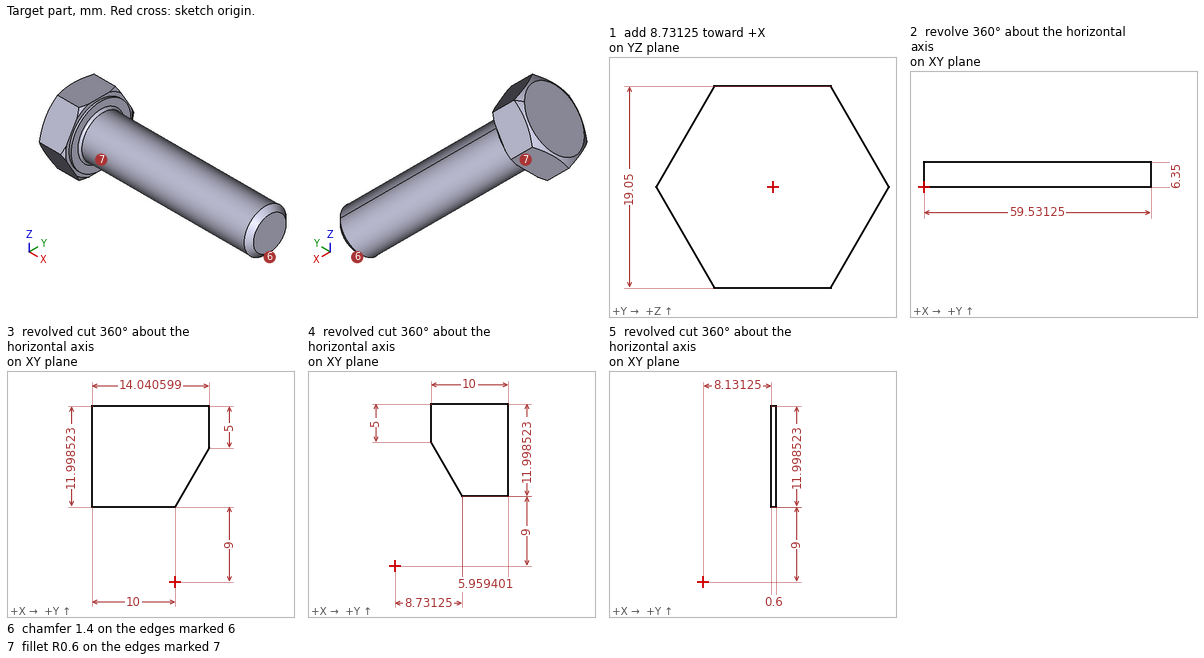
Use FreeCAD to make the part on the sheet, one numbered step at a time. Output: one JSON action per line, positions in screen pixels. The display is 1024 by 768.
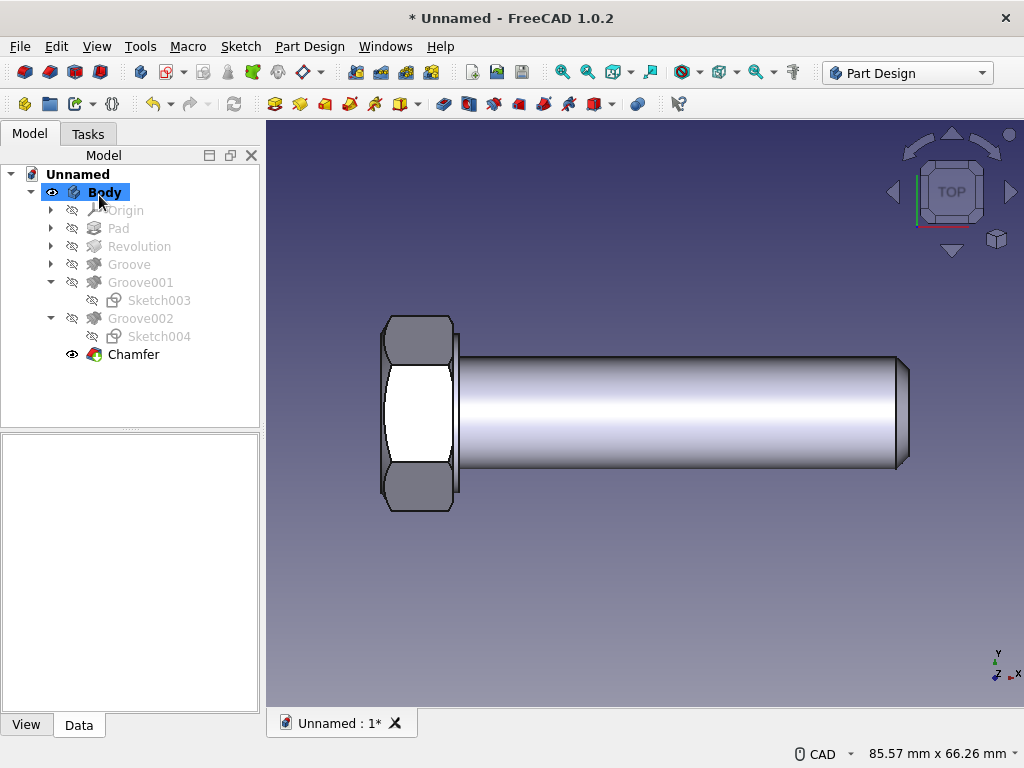
{"action": "key", "text": "1"}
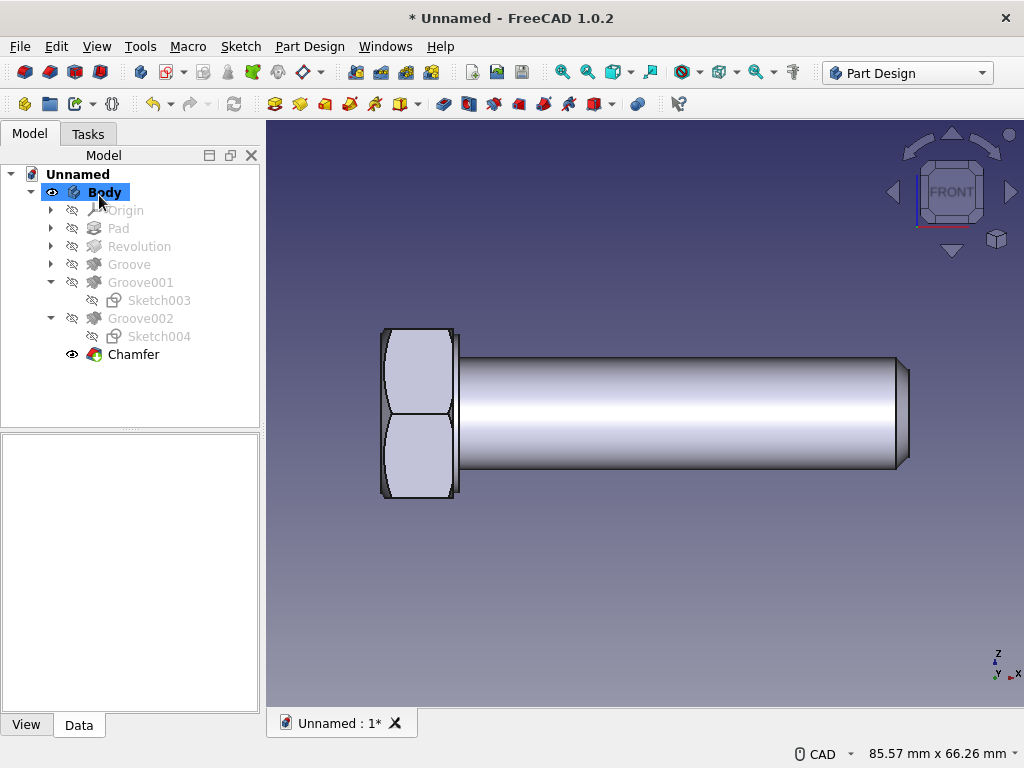
{"action": "key", "text": "3"}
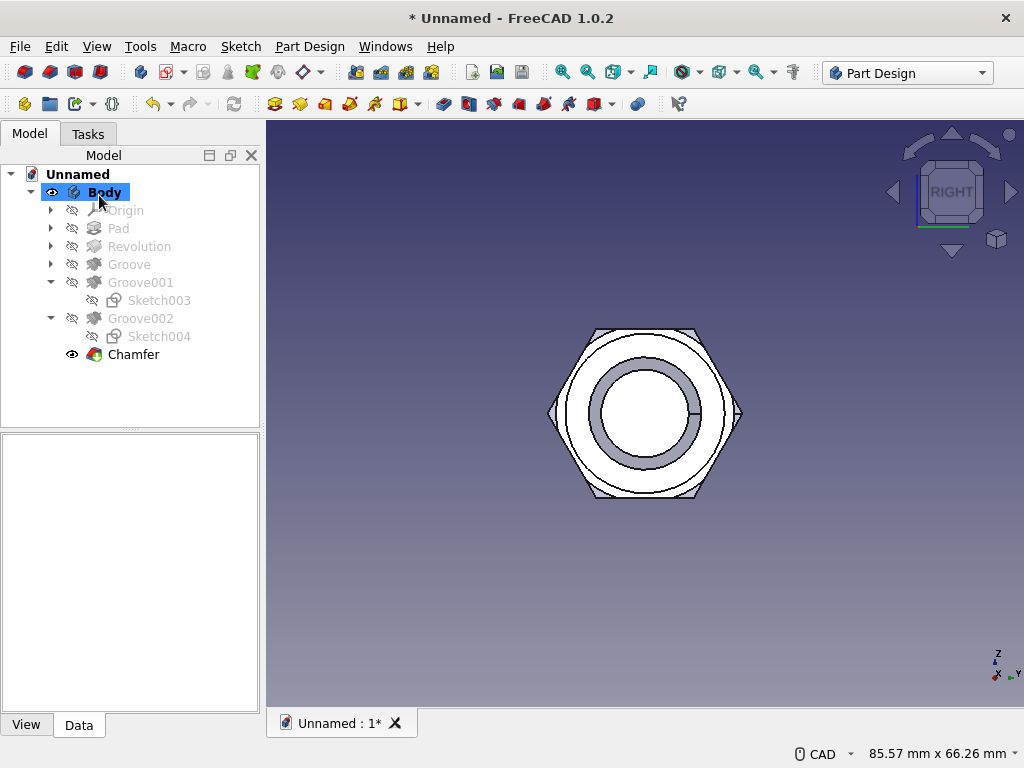
{"action": "left_click", "coordinate": [563, 72]}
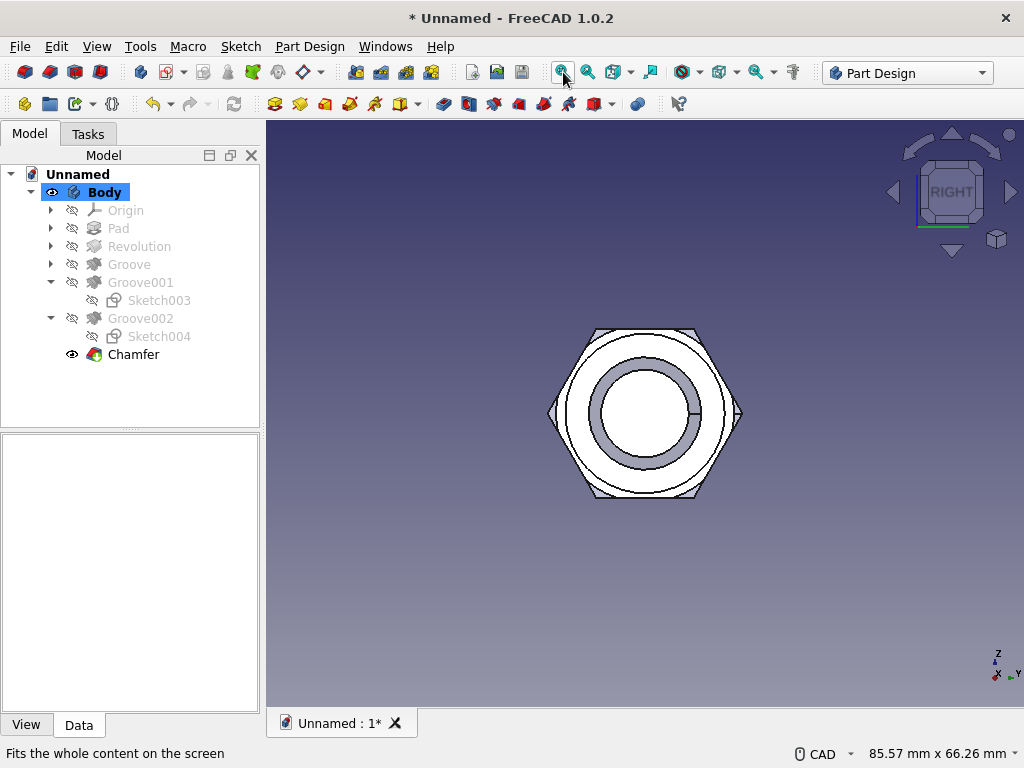
{"action": "key", "text": "5"}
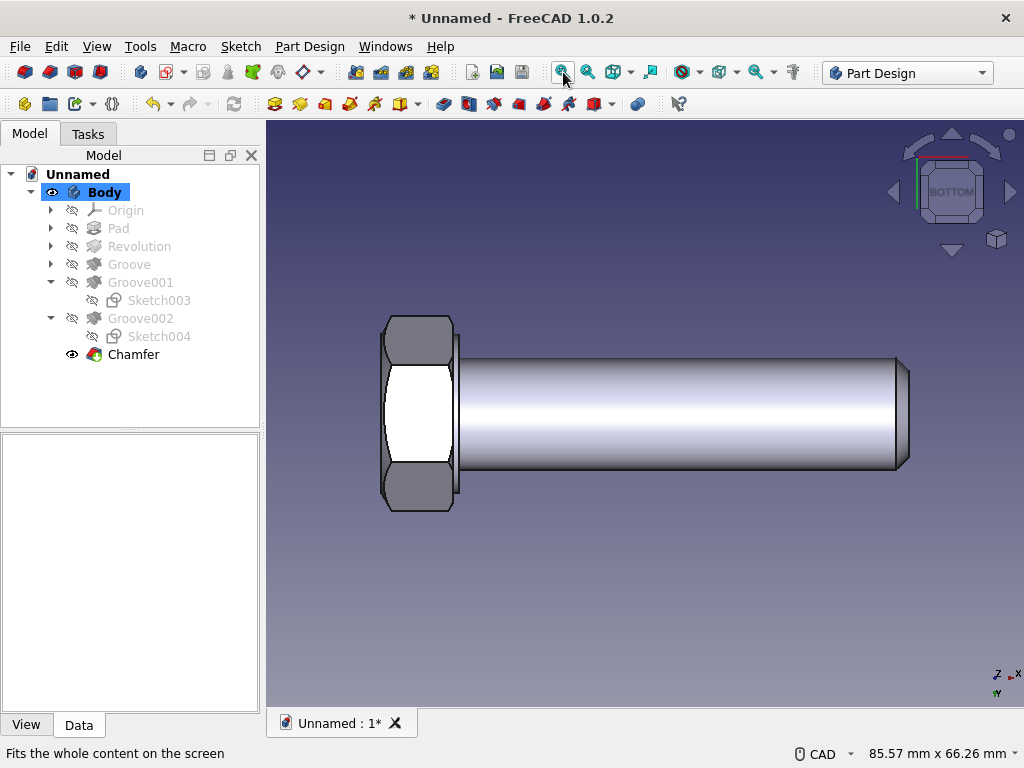
{"action": "key", "text": "4"}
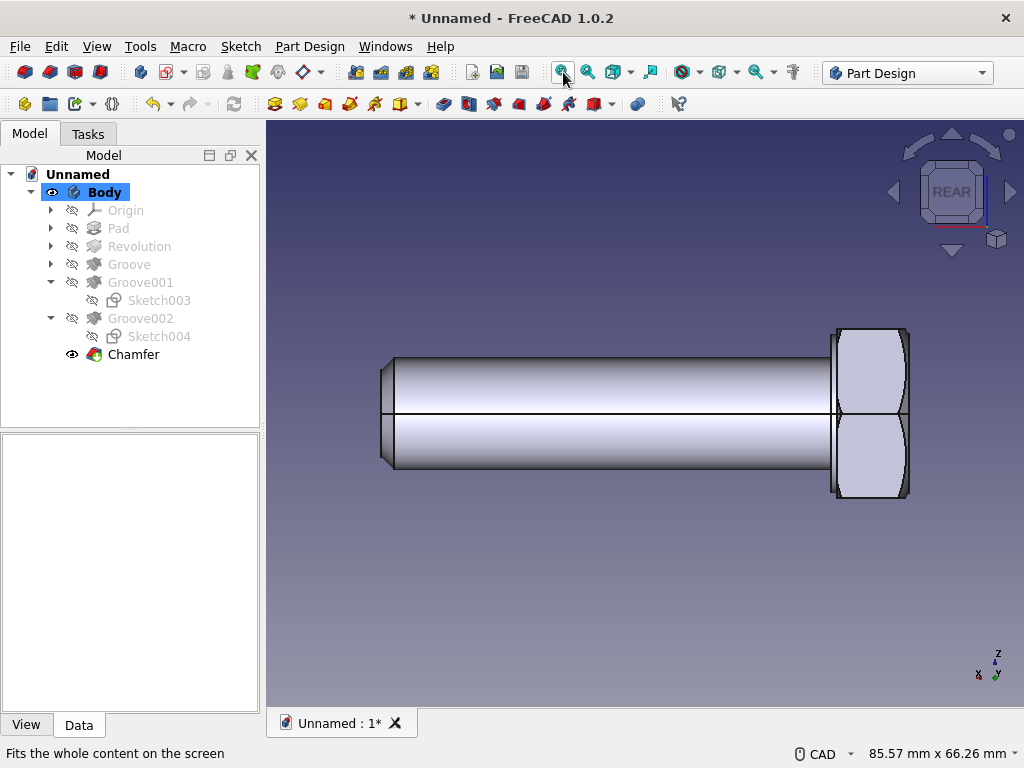
{"action": "key", "text": "6"}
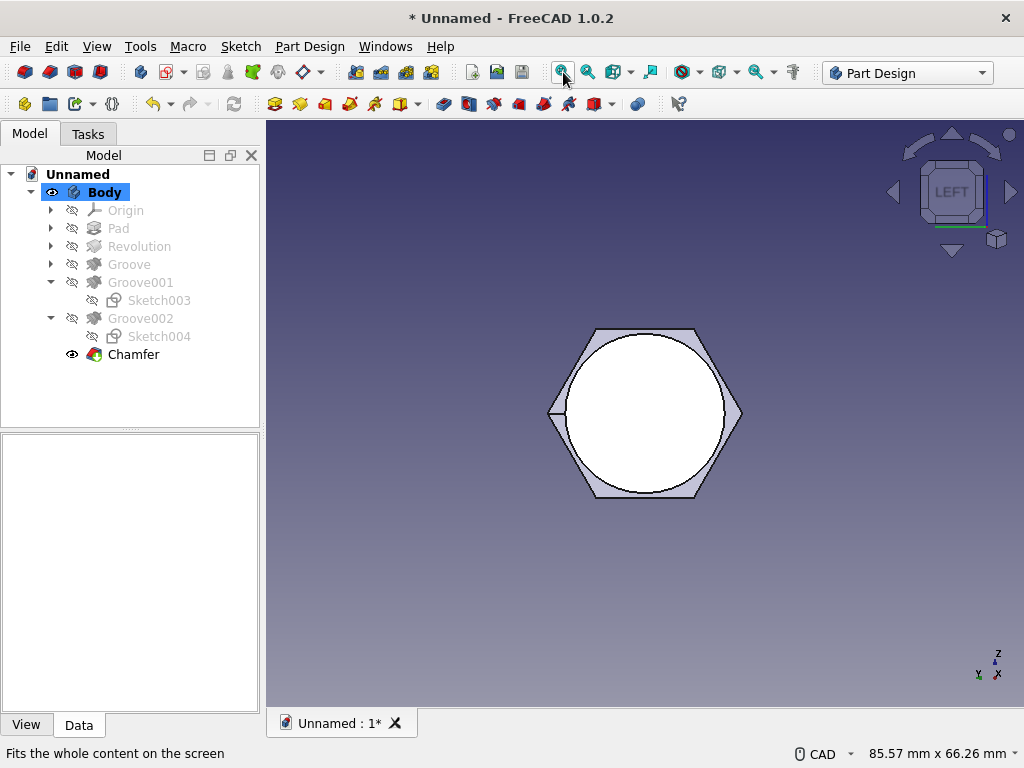
{"action": "left_click", "coordinate": [563, 72]}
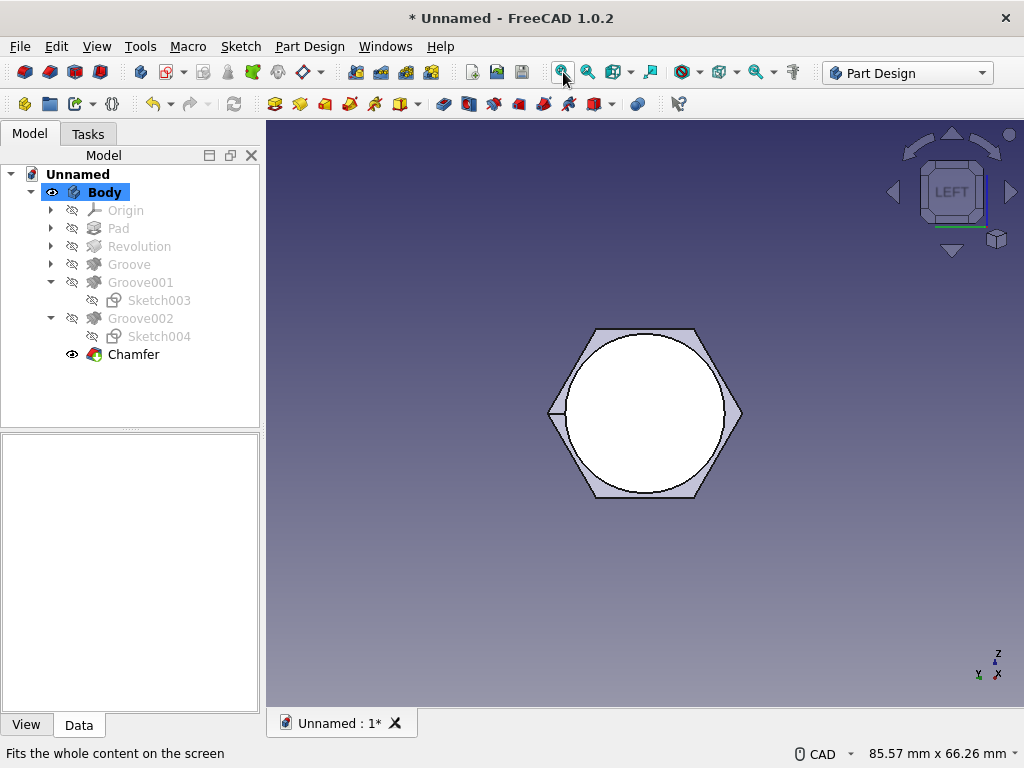
{"action": "key", "text": "v 3"}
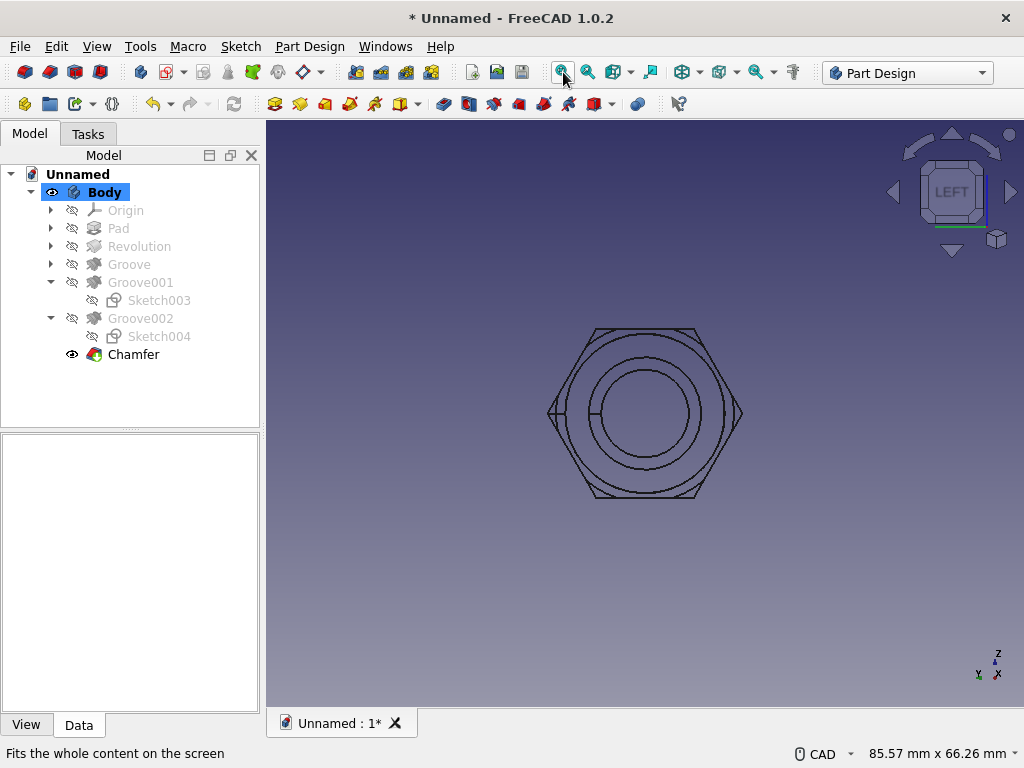
{"action": "key", "text": "0"}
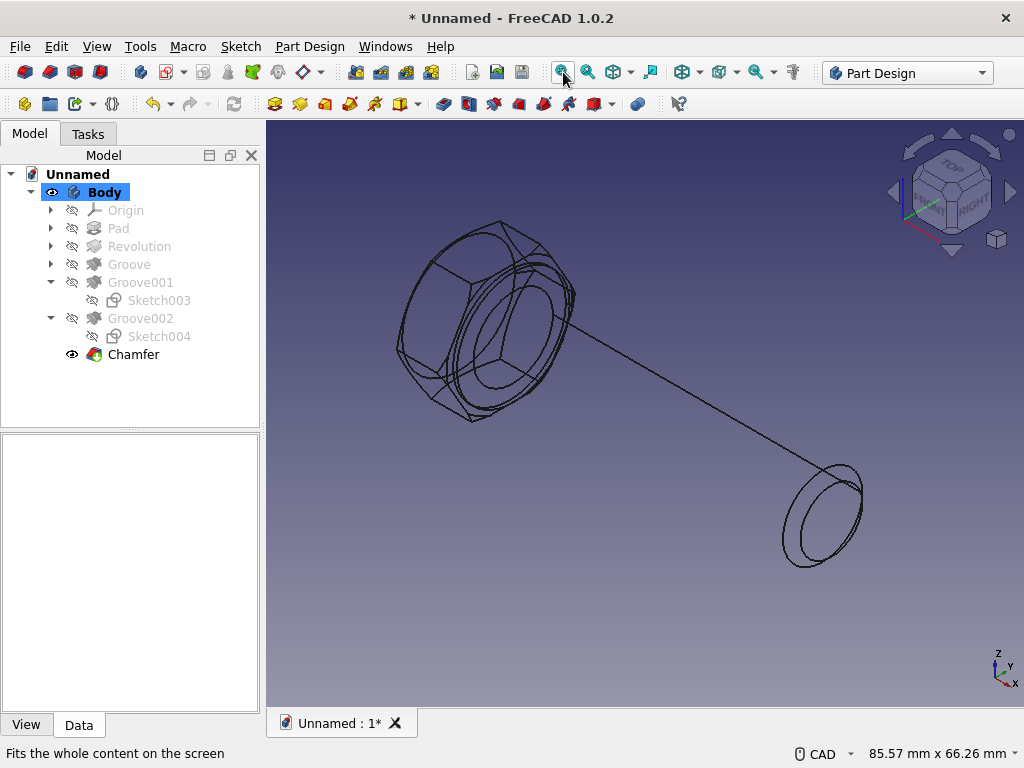
{"action": "left_click", "coordinate": [473, 359]}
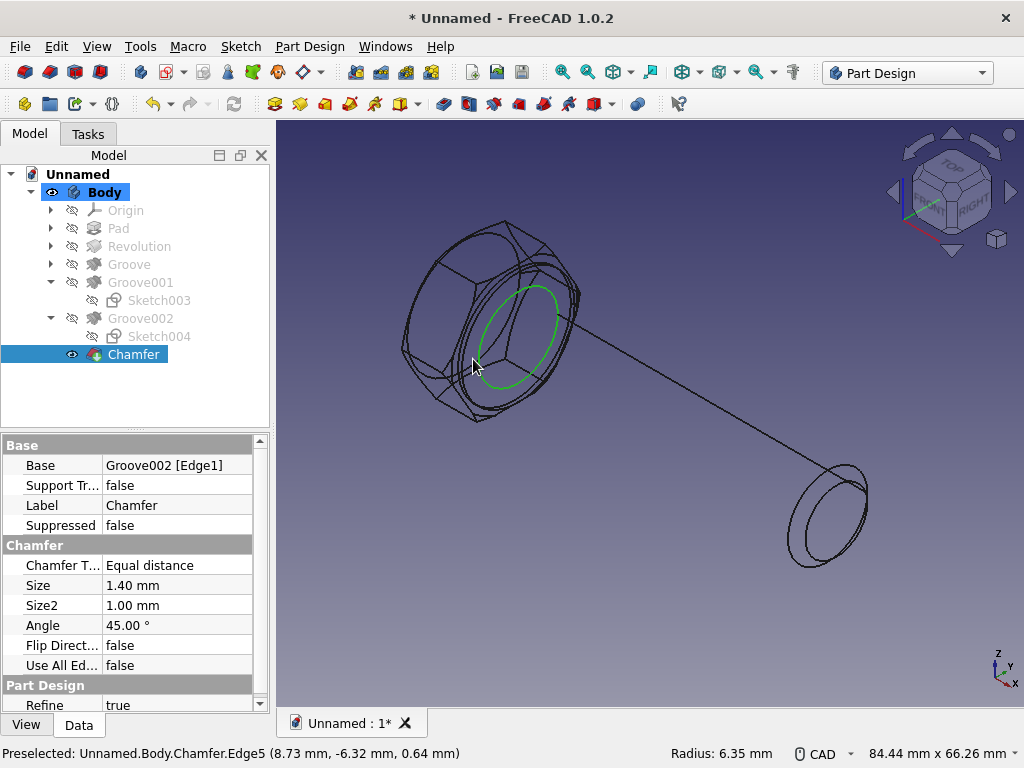
{"action": "key", "text": "v 1"}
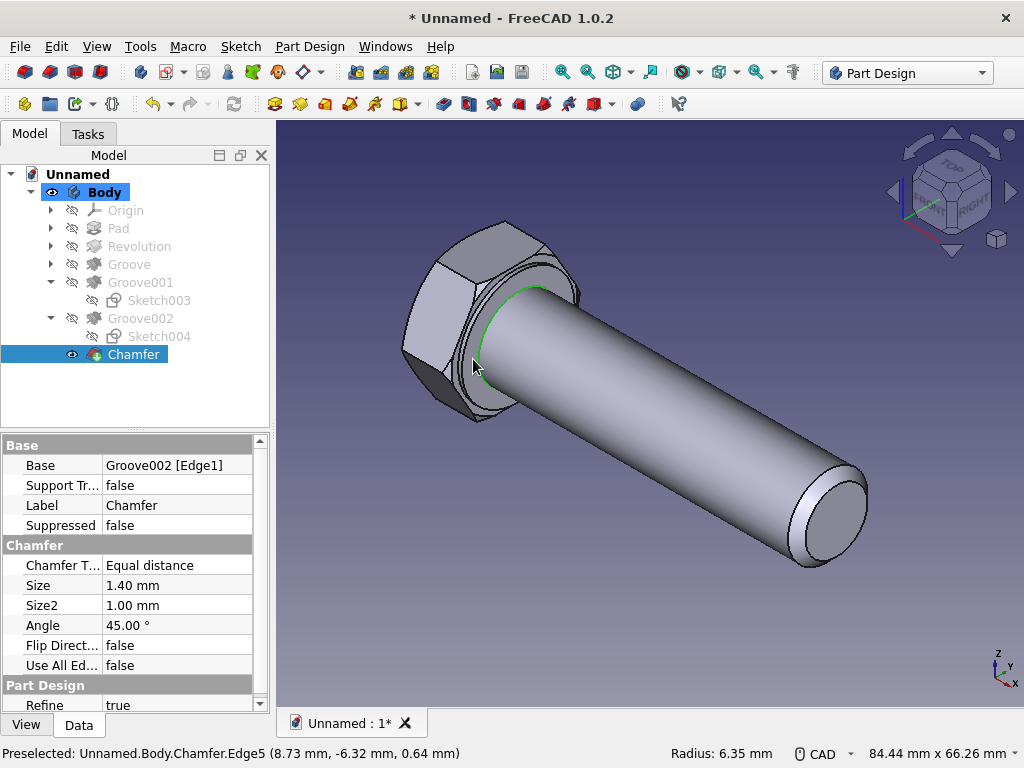
{"action": "left_click", "coordinate": [25, 72]}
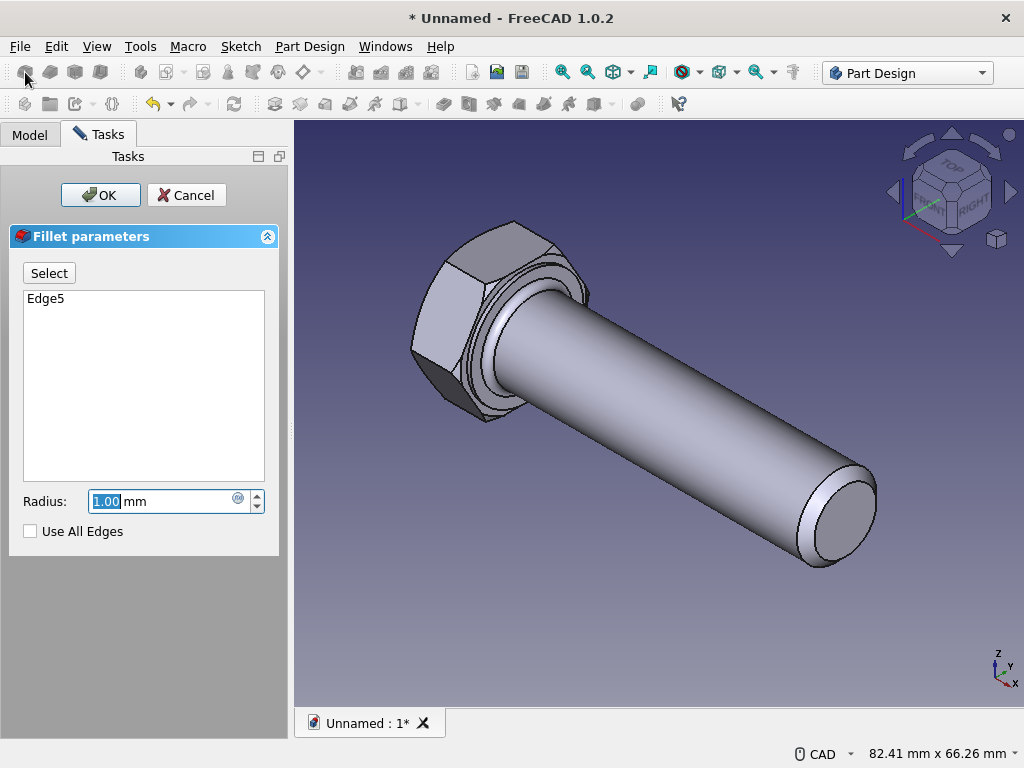
{"action": "type", "text": "0.6"}
{"action": "key", "text": "Tab"}